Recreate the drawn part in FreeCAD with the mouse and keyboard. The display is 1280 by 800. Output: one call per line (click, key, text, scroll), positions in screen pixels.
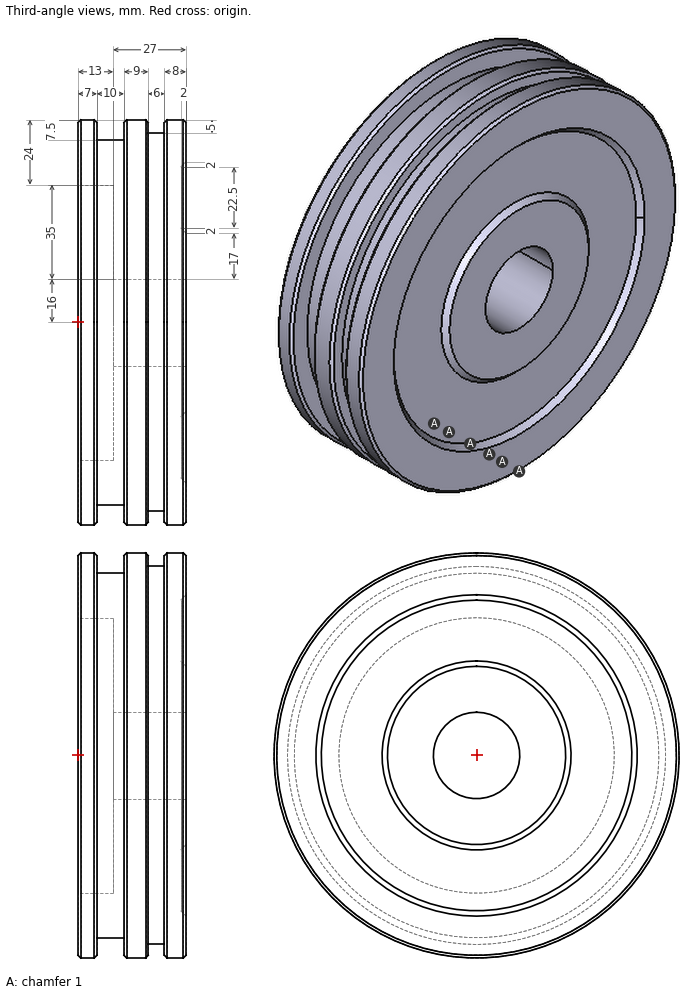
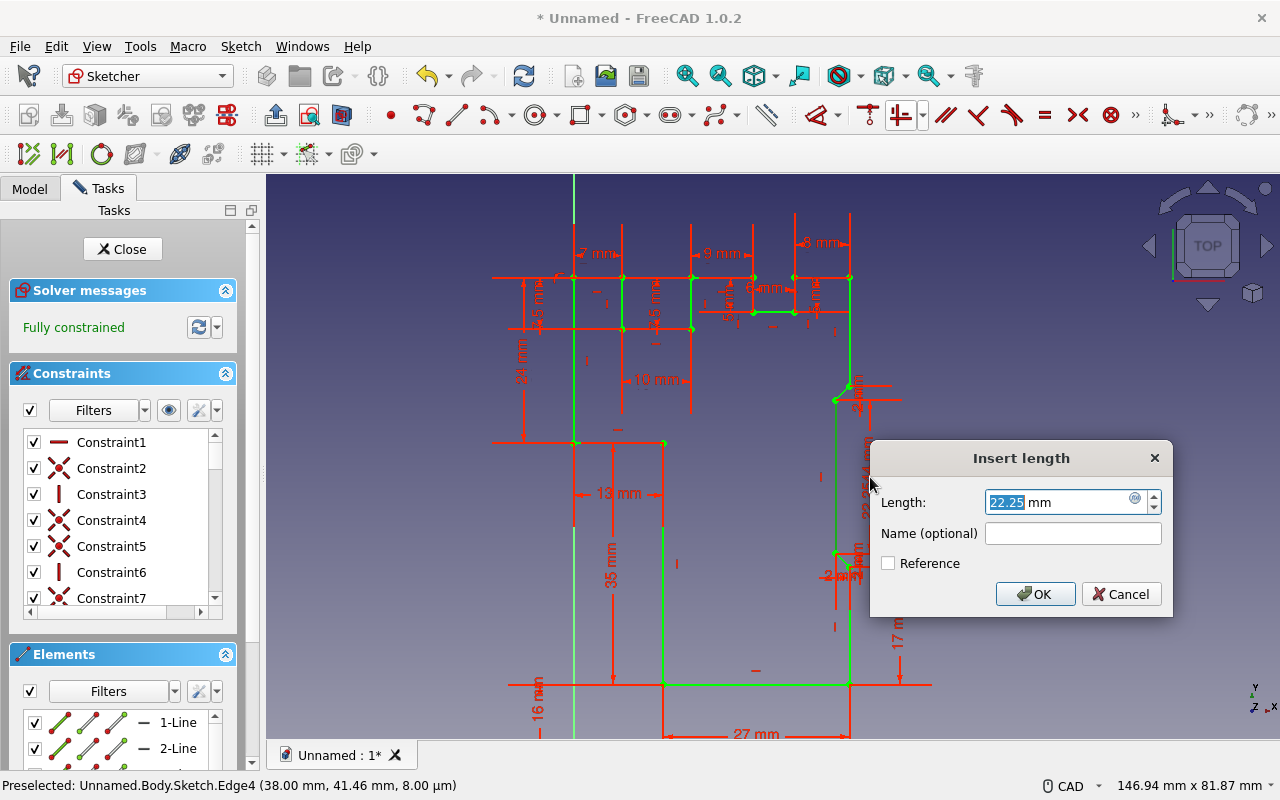
text(22.5)
key(Return)
key(Escape)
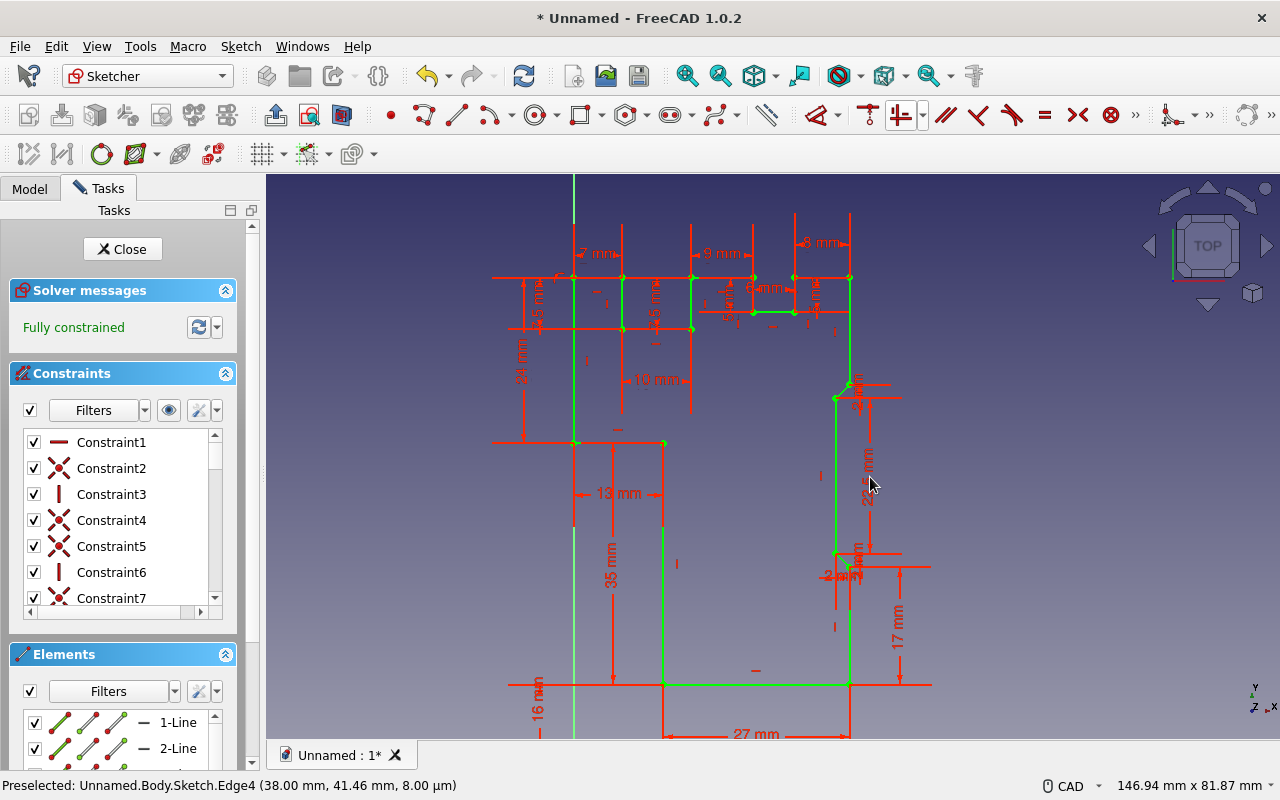
click(123, 249)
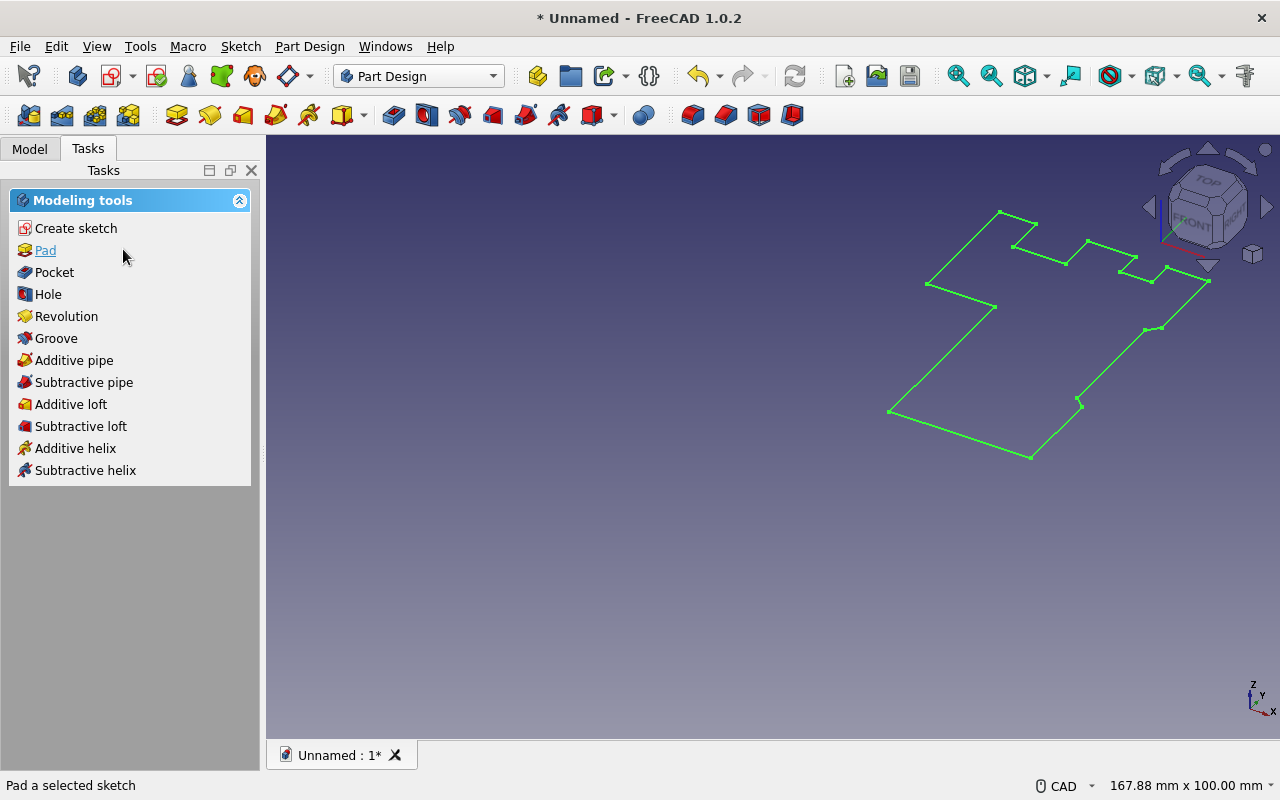
click(210, 116)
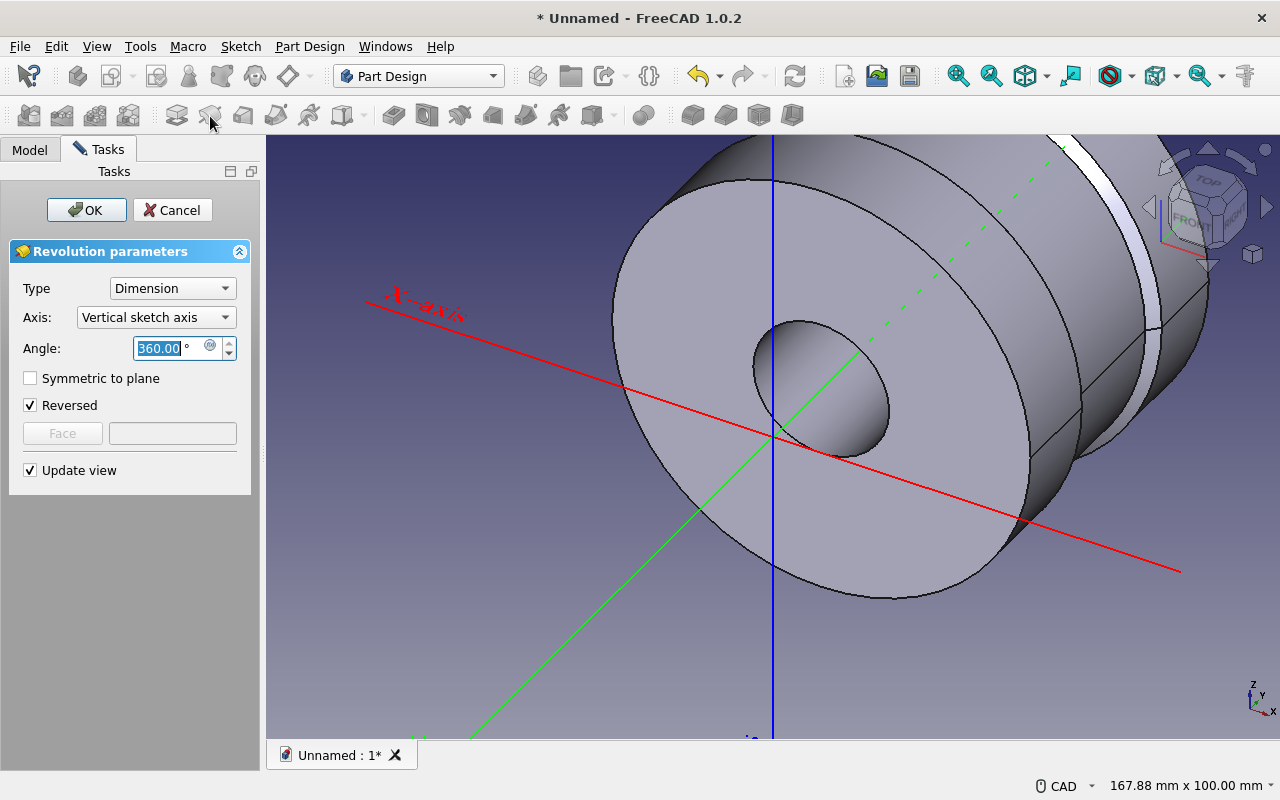
click(157, 318)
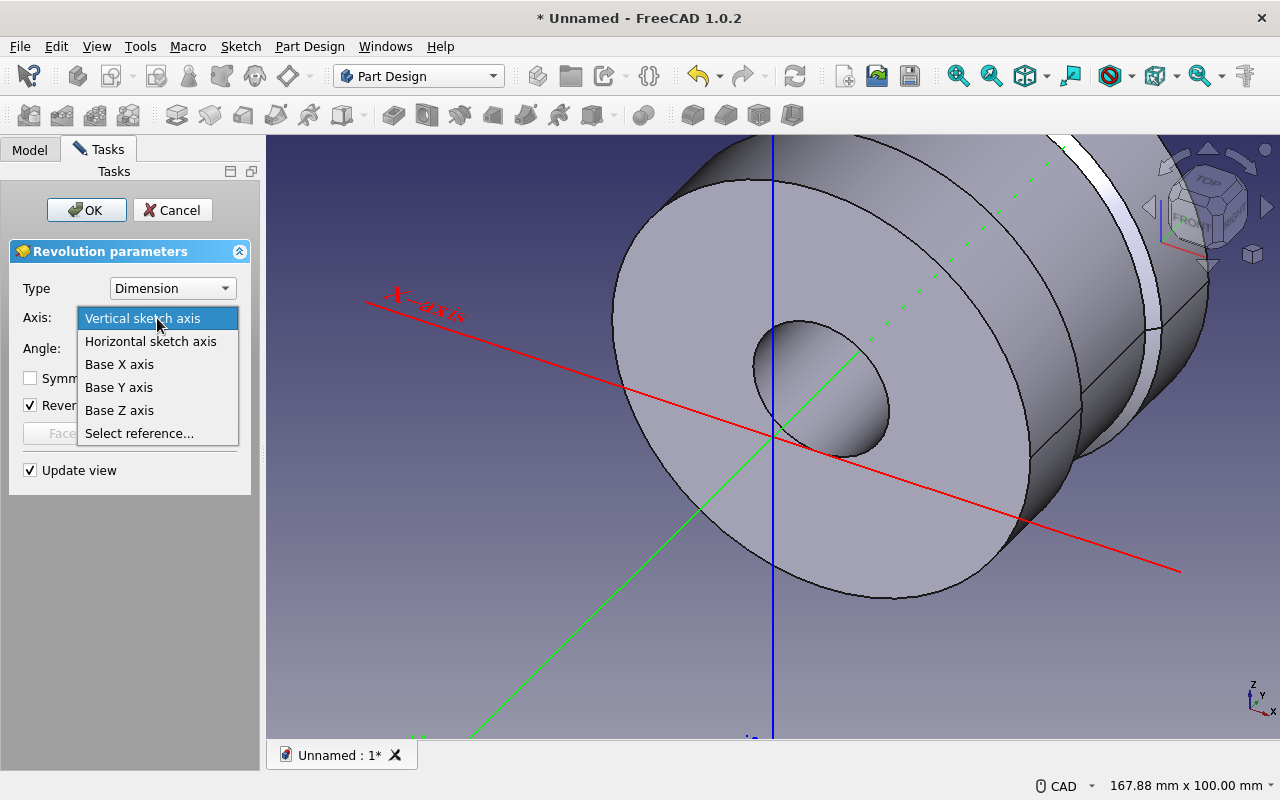
click(156, 342)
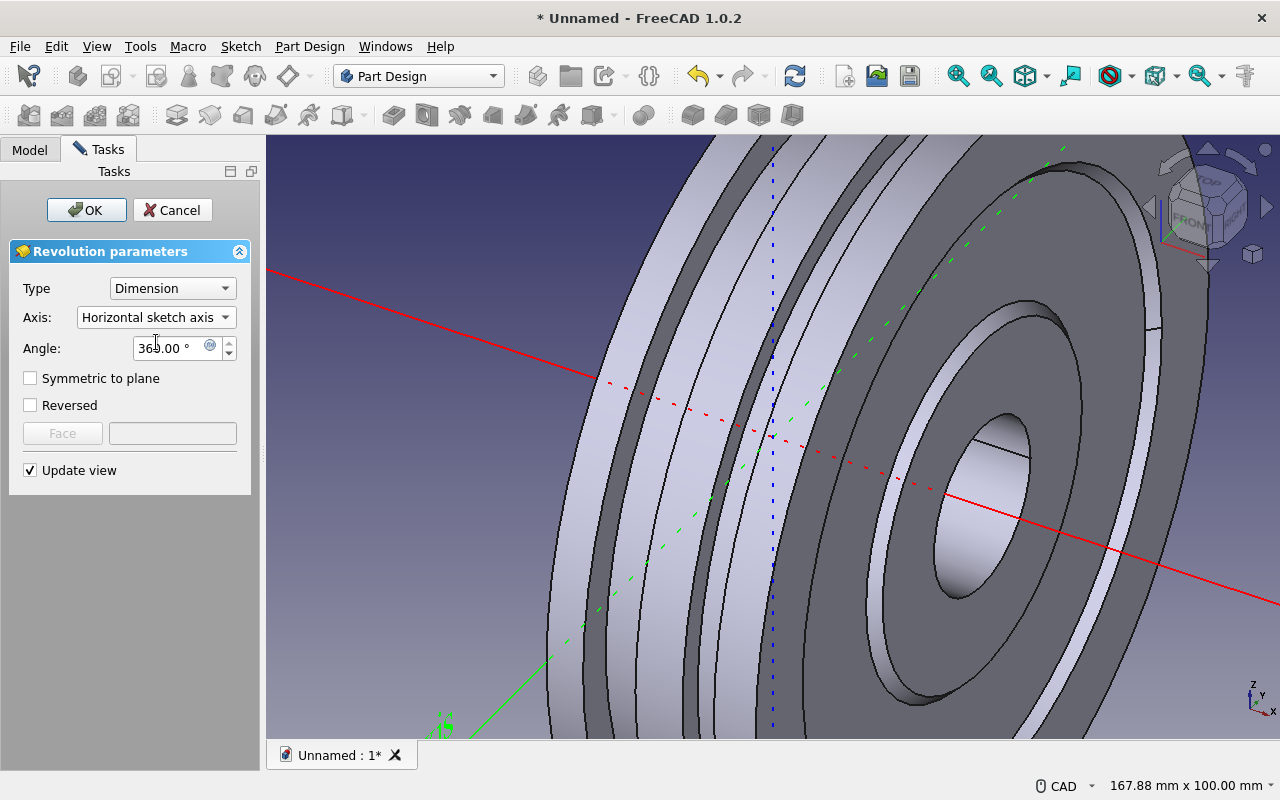
click(87, 210)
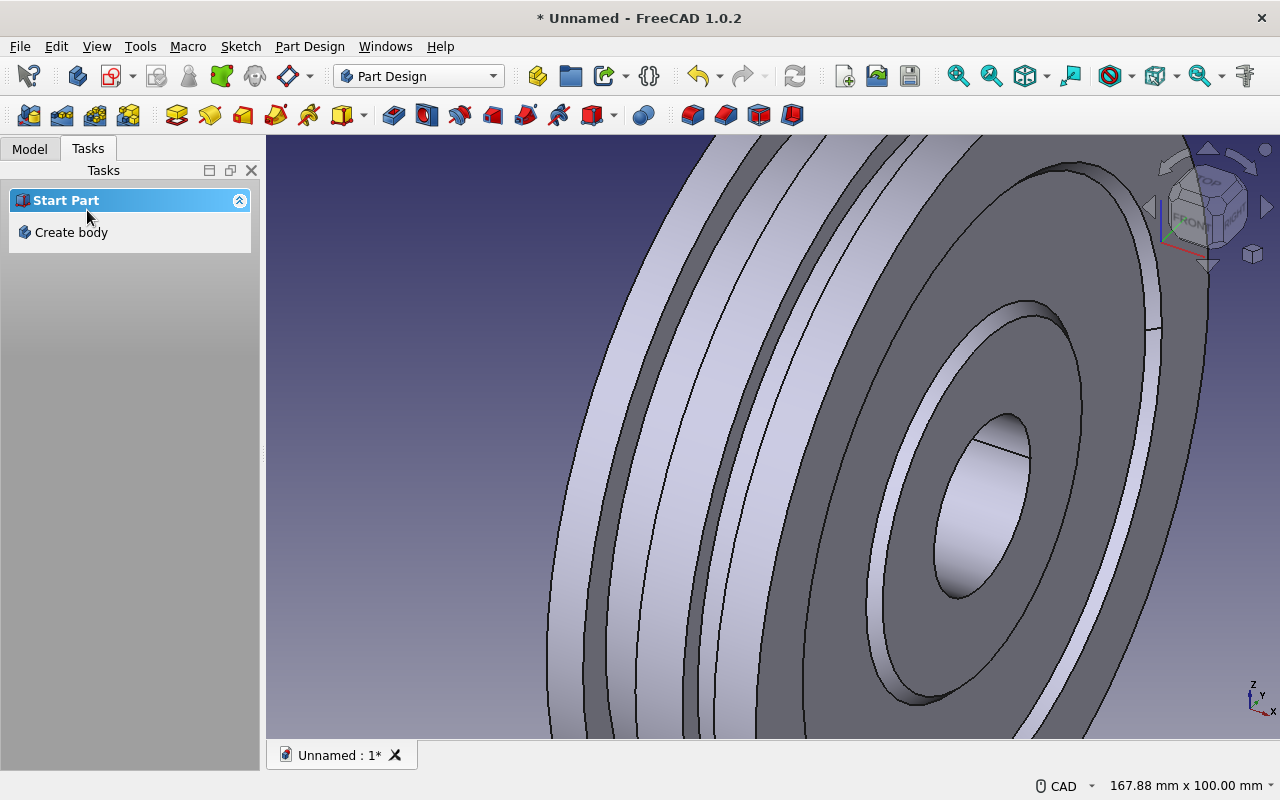
click(959, 76)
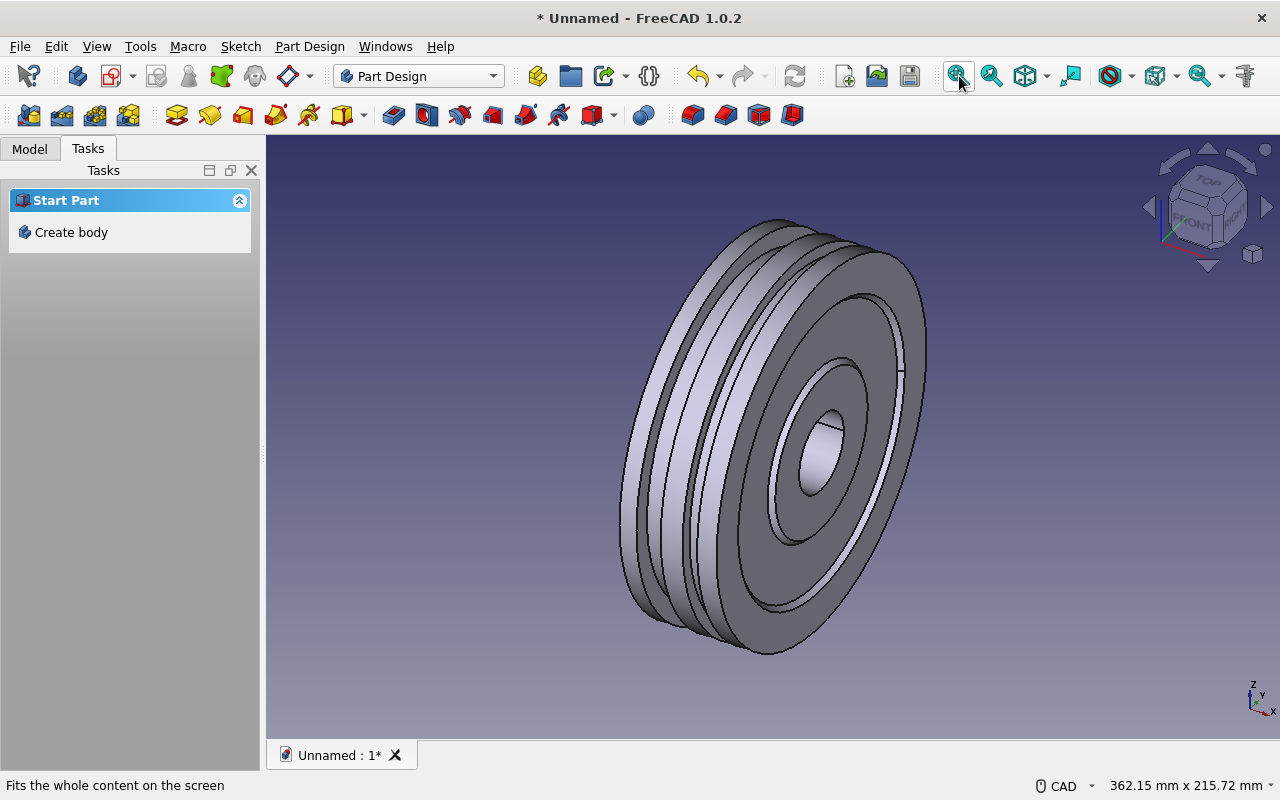
click(716, 556)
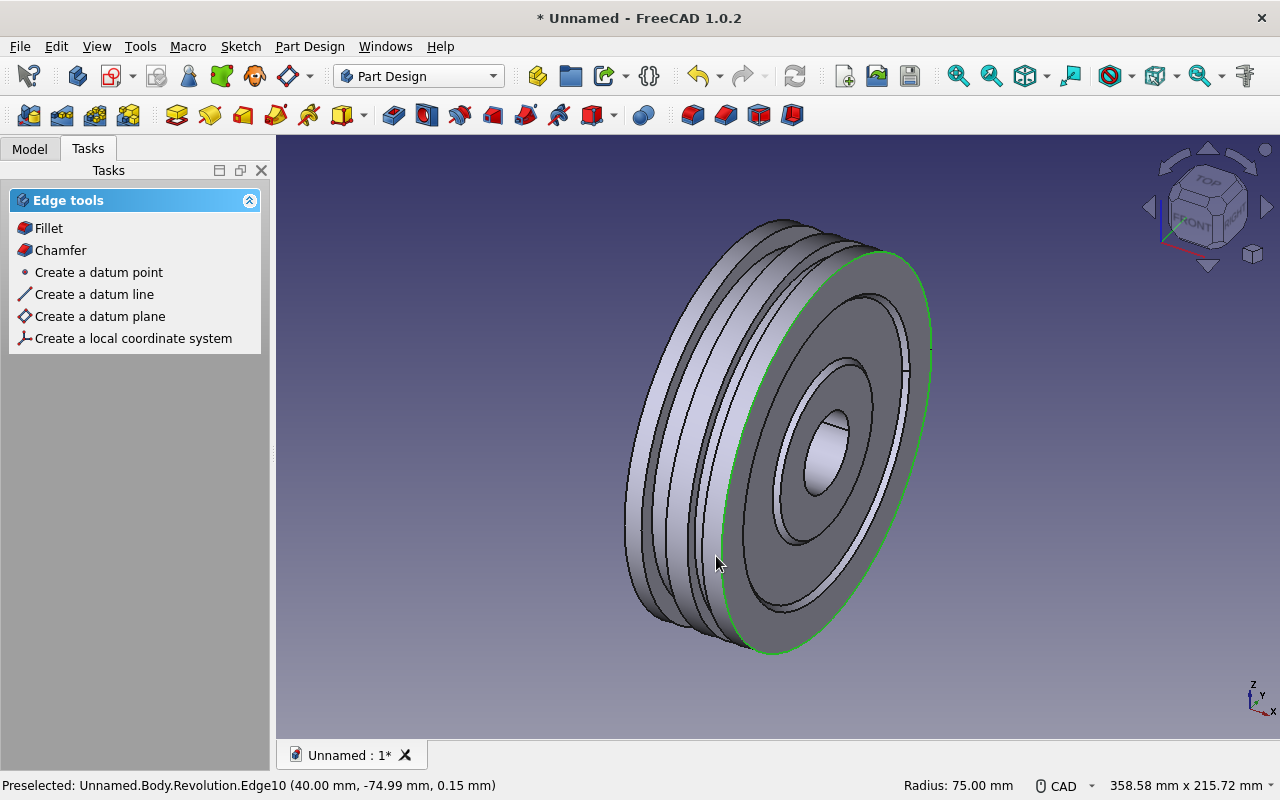
click(688, 545, ctrl)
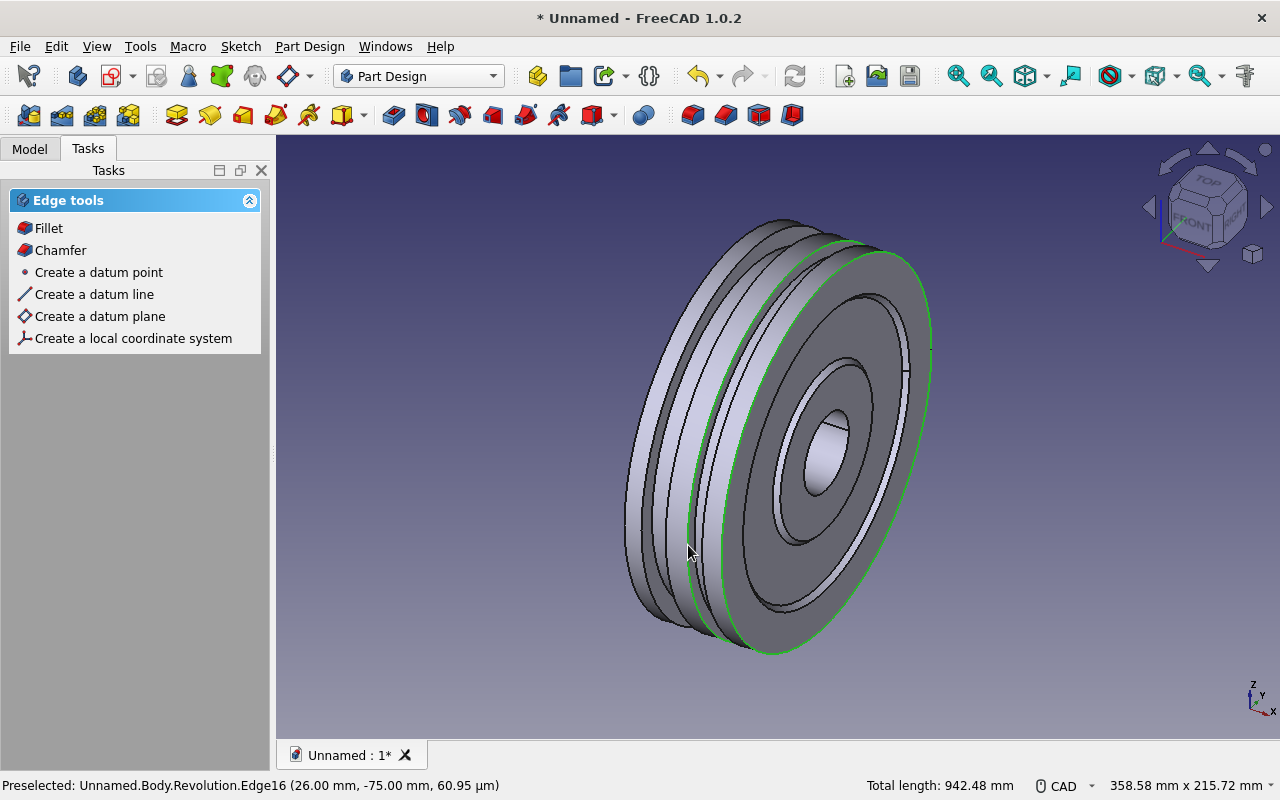
click(641, 530, ctrl)